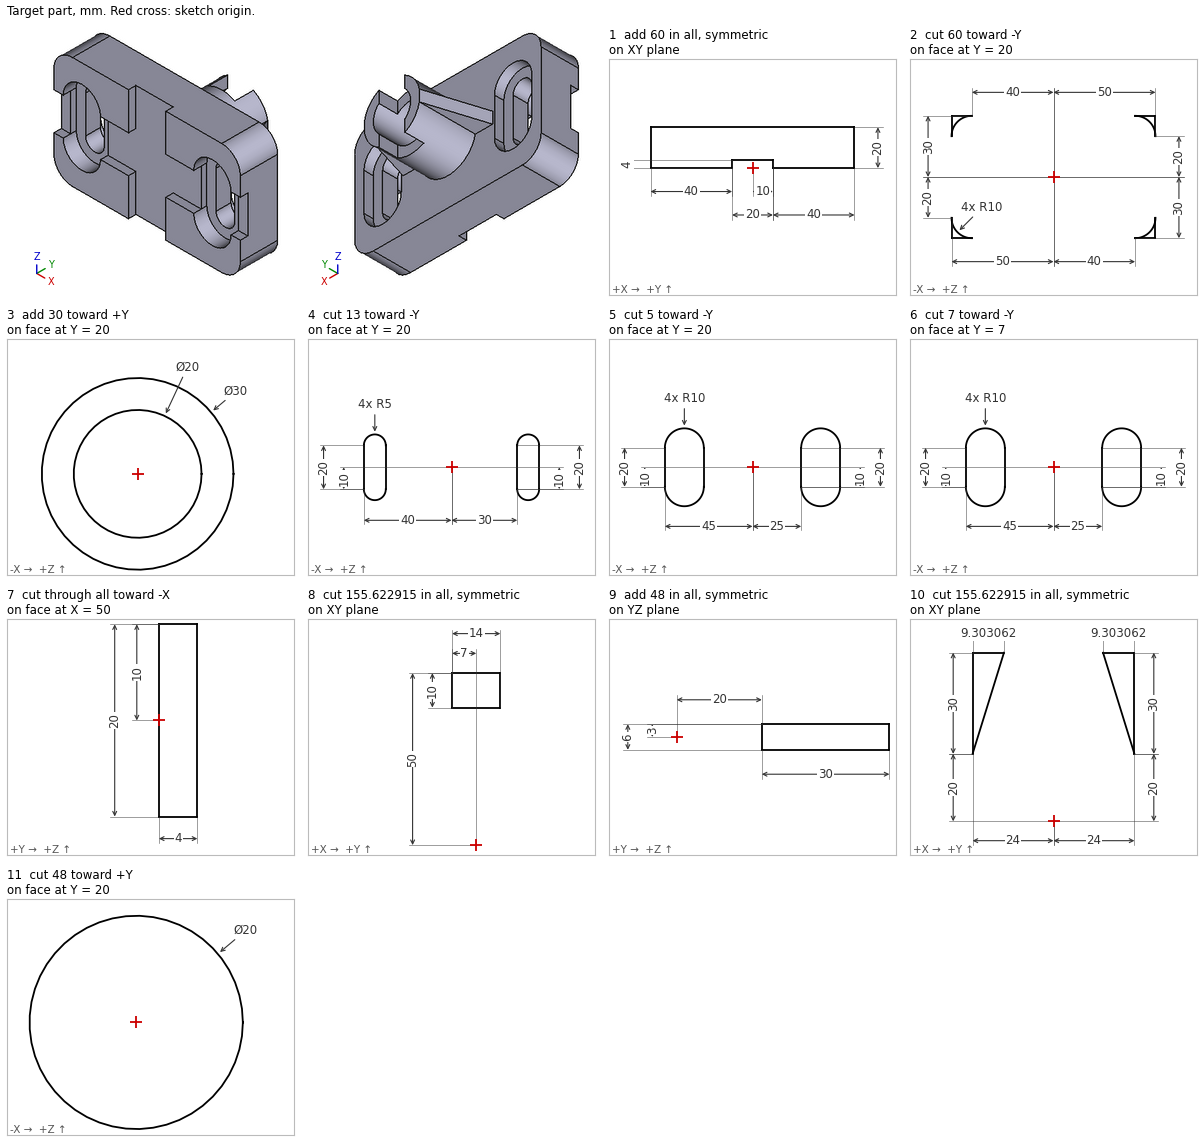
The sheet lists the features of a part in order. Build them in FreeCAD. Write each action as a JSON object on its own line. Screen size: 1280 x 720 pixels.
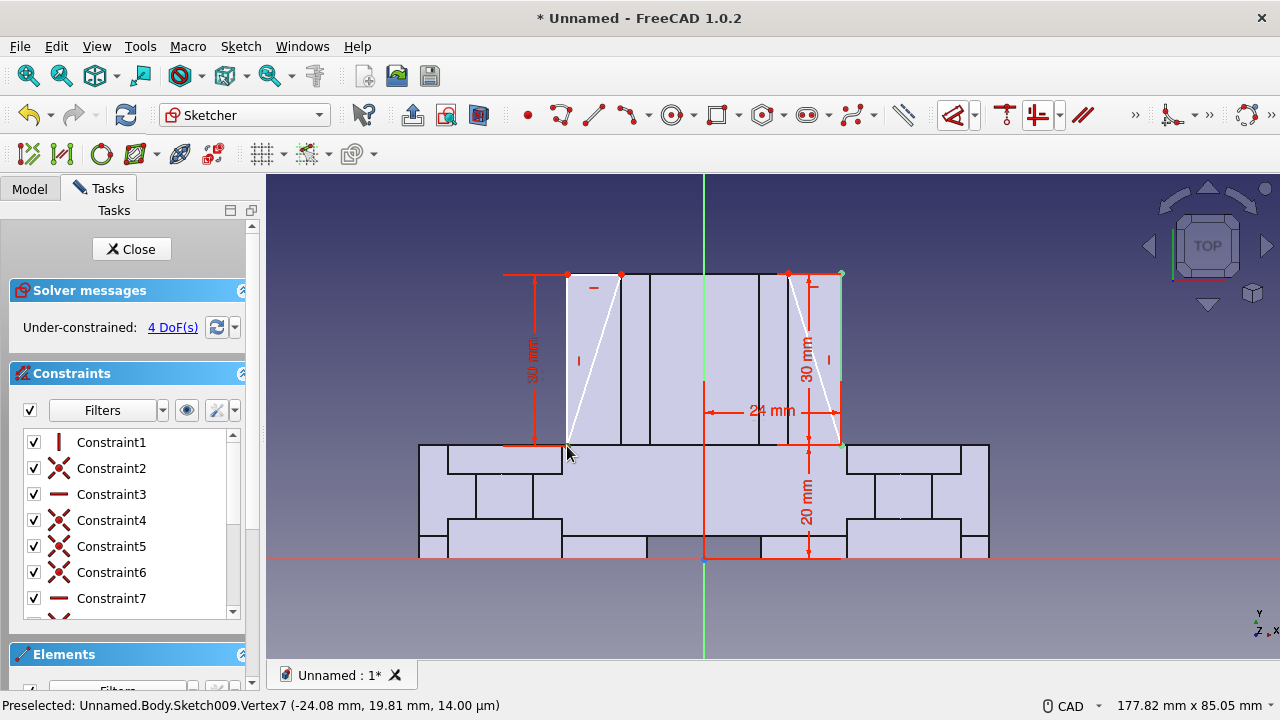
{"action": "key", "text": "l"}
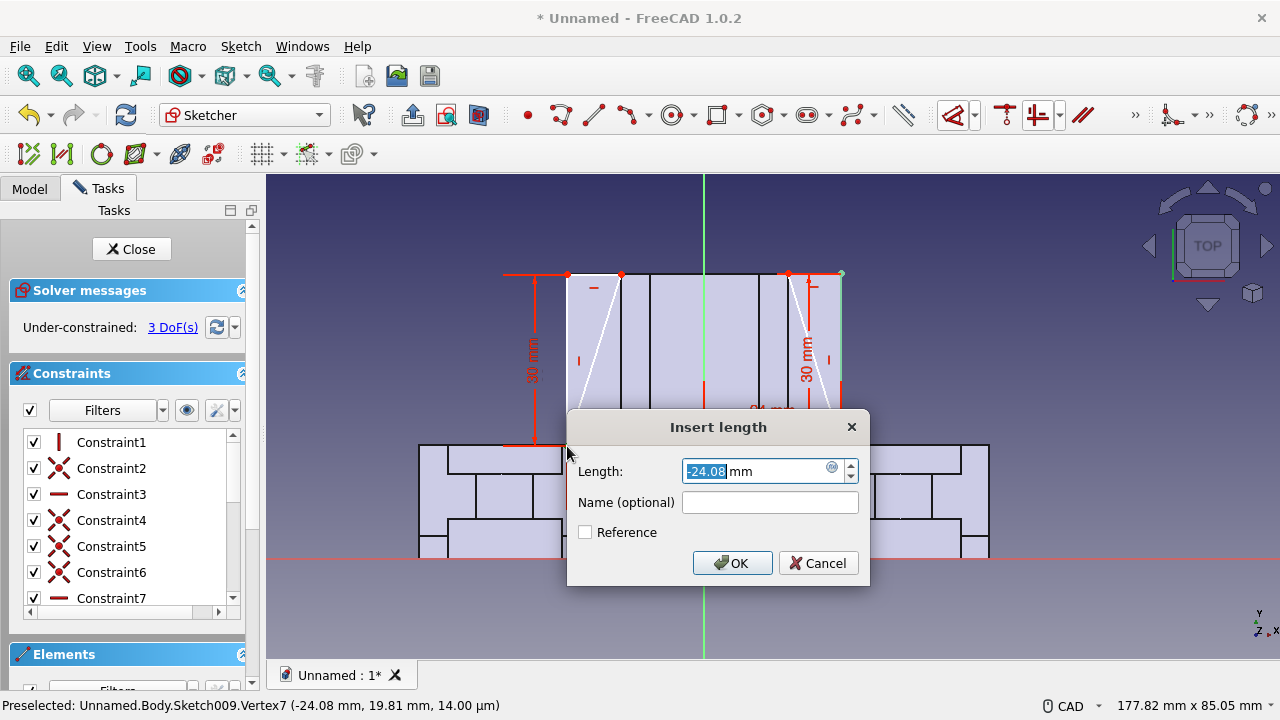
{"action": "type", "text": "-24"}
{"action": "key", "text": "Return"}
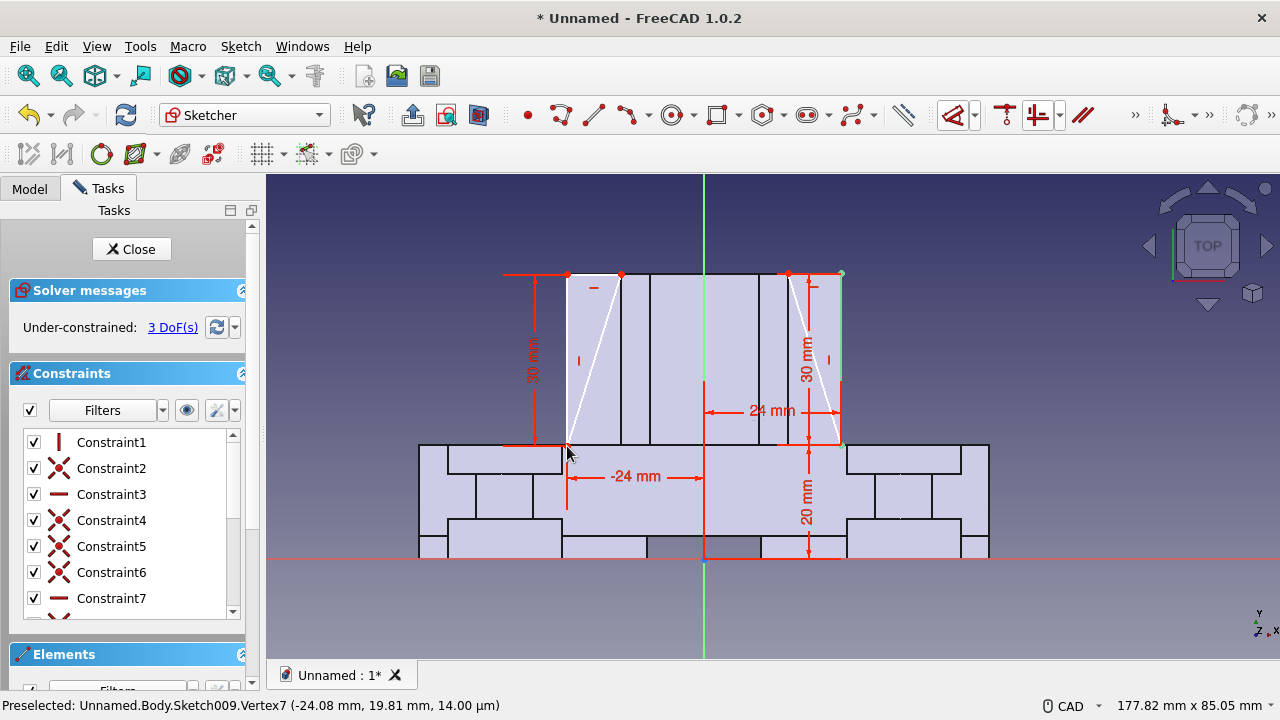
{"action": "left_click", "coordinate": [567, 446]}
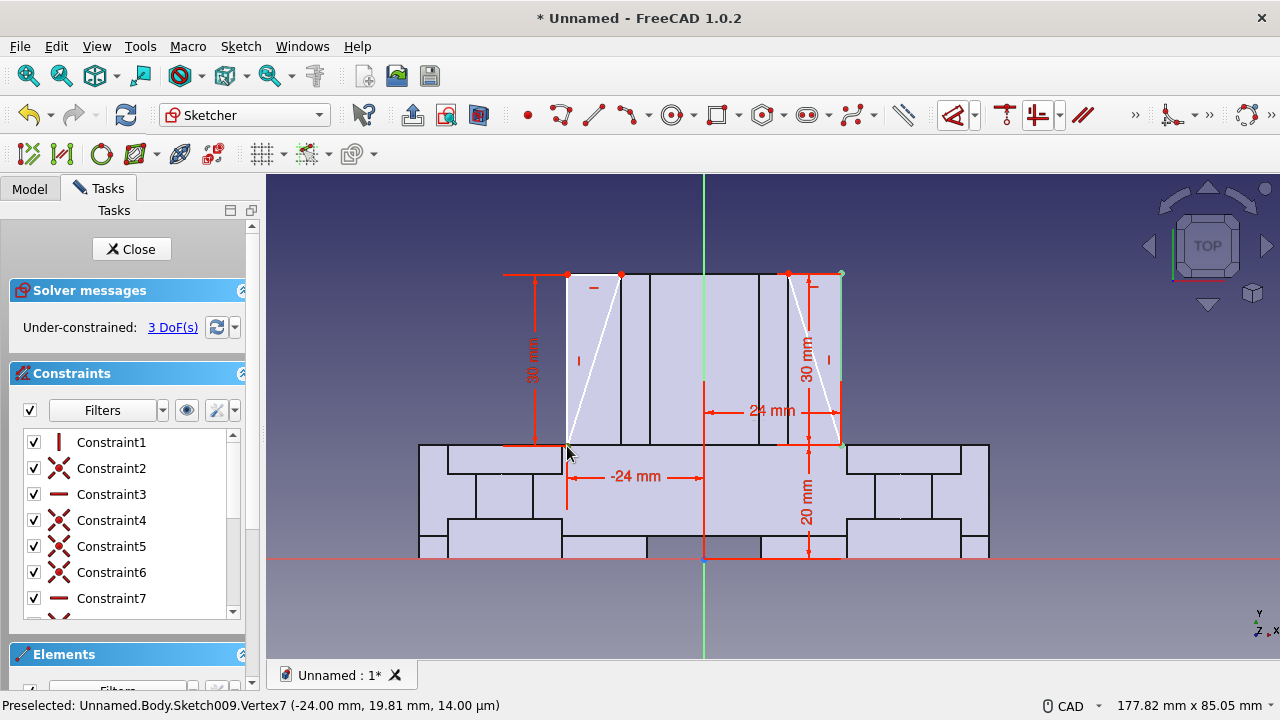
{"action": "key", "text": "i"}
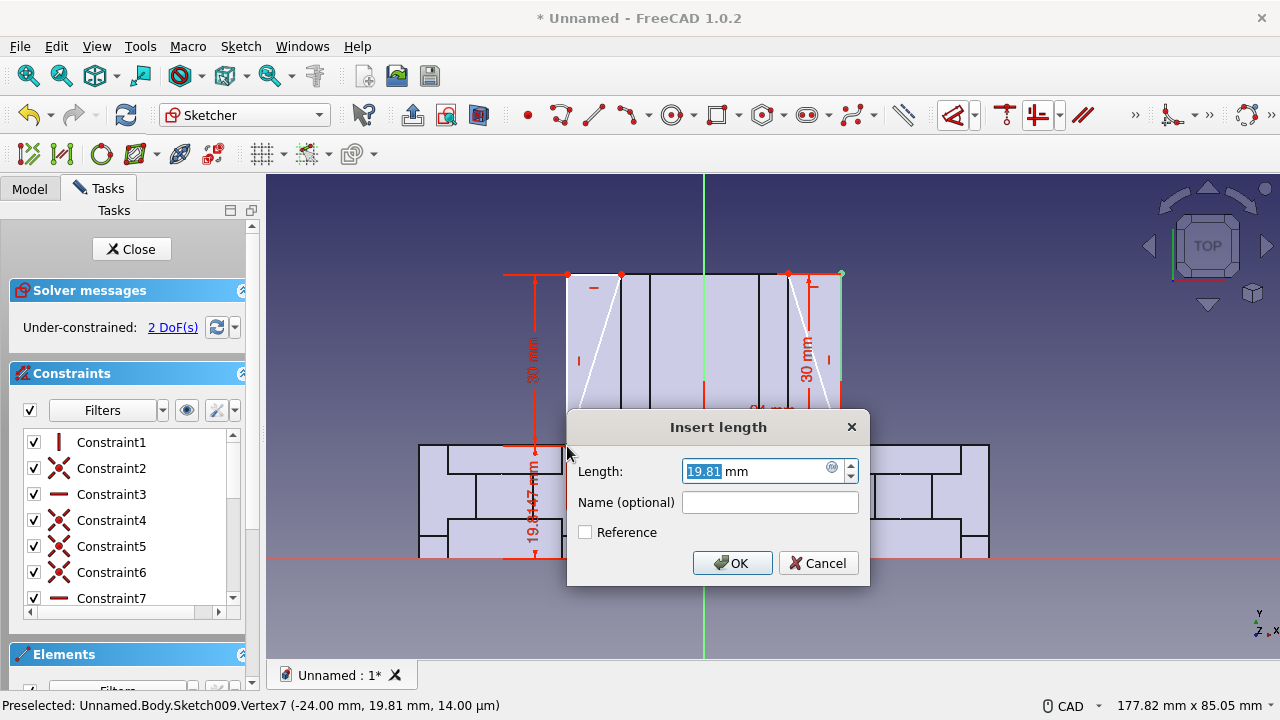
{"action": "type", "text": "20"}
{"action": "key", "text": "Return"}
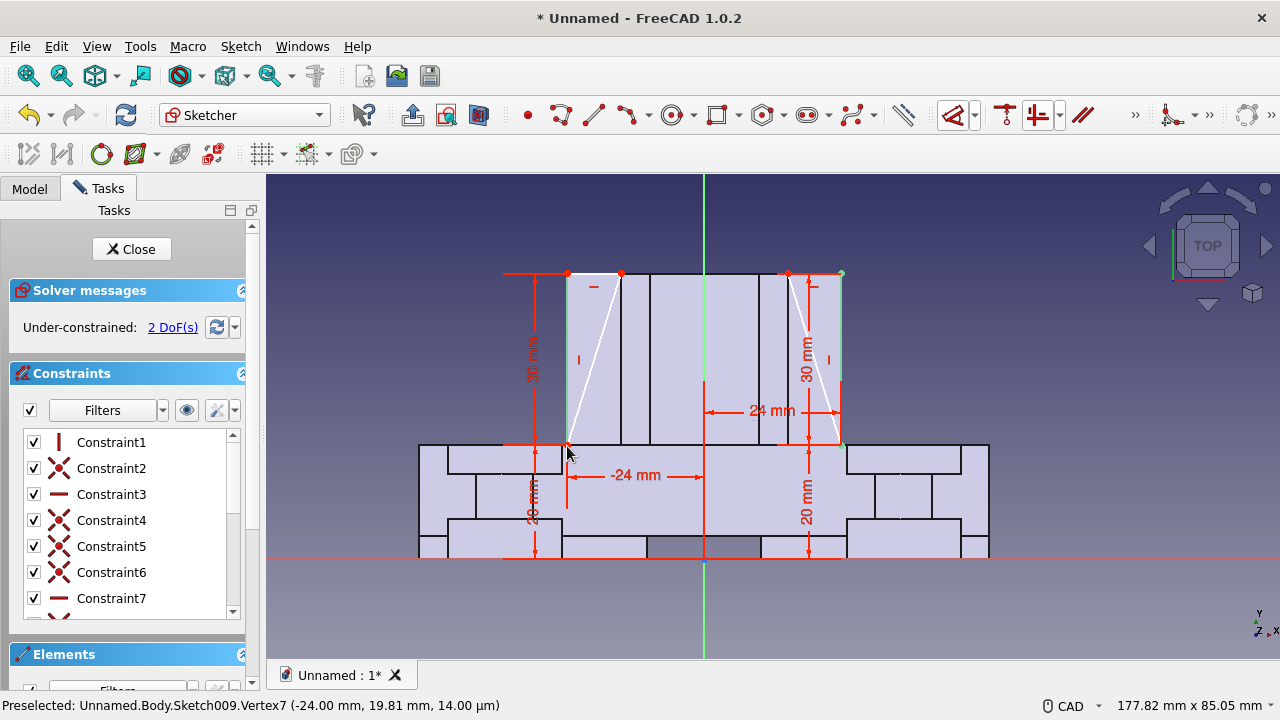
{"action": "left_click", "coordinate": [825, 274]}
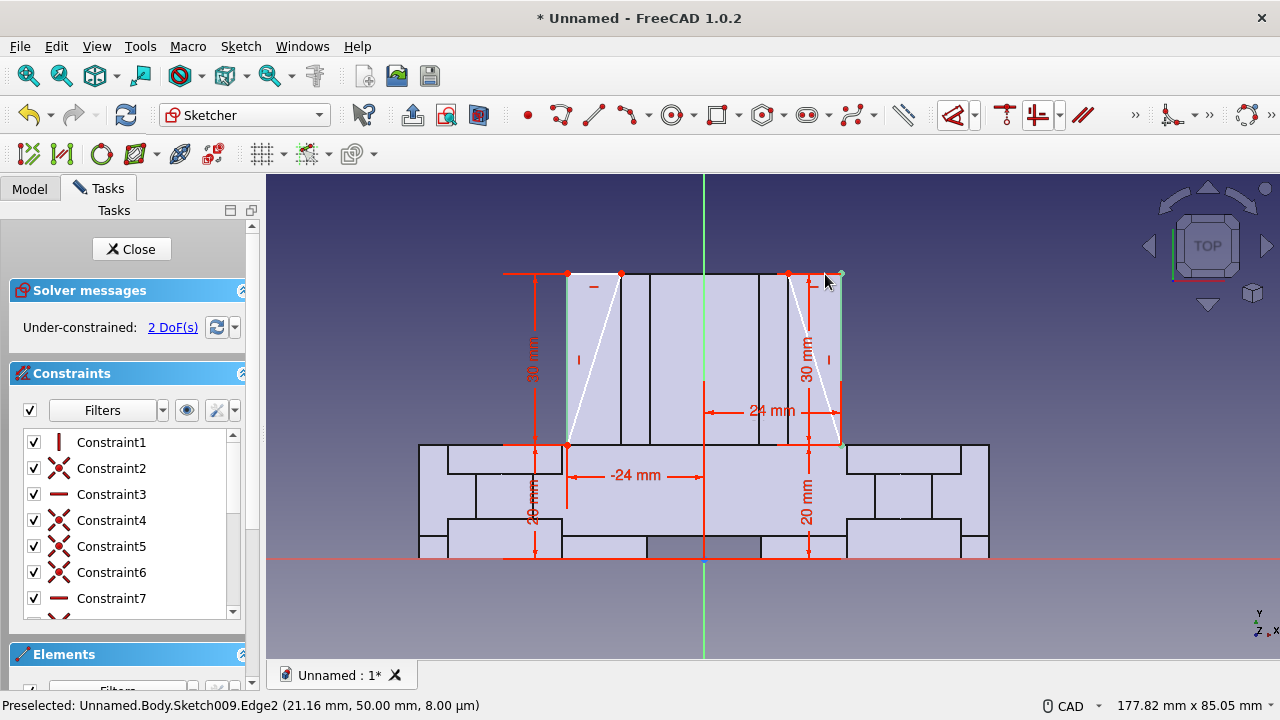
{"action": "key", "text": "l"}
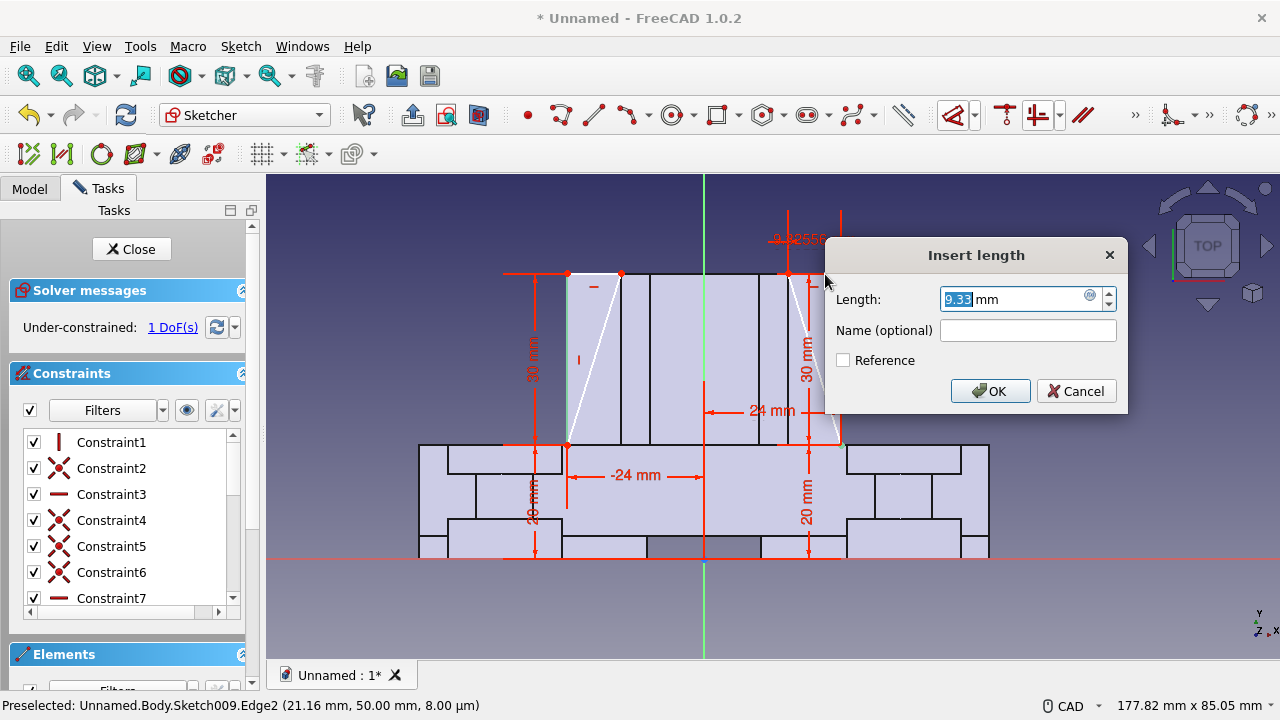
{"action": "type", "text": "9.303062"}
{"action": "key", "text": "Return"}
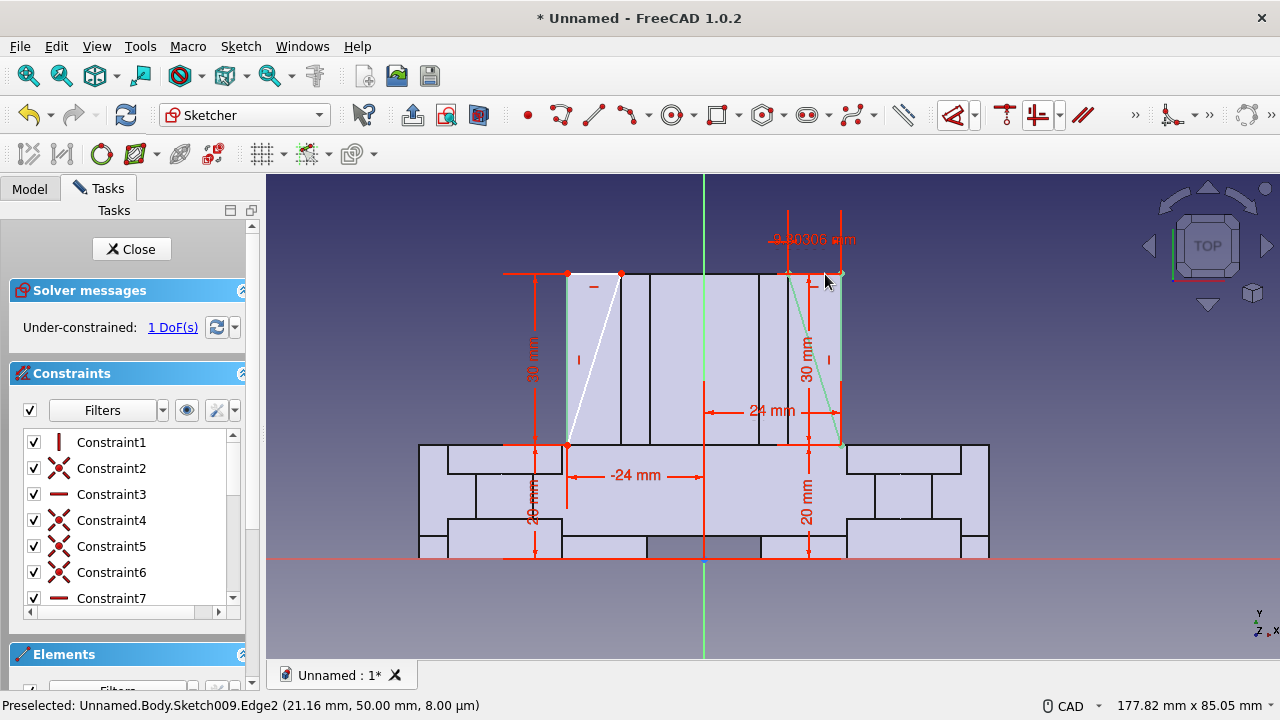
{"action": "left_click", "coordinate": [605, 274]}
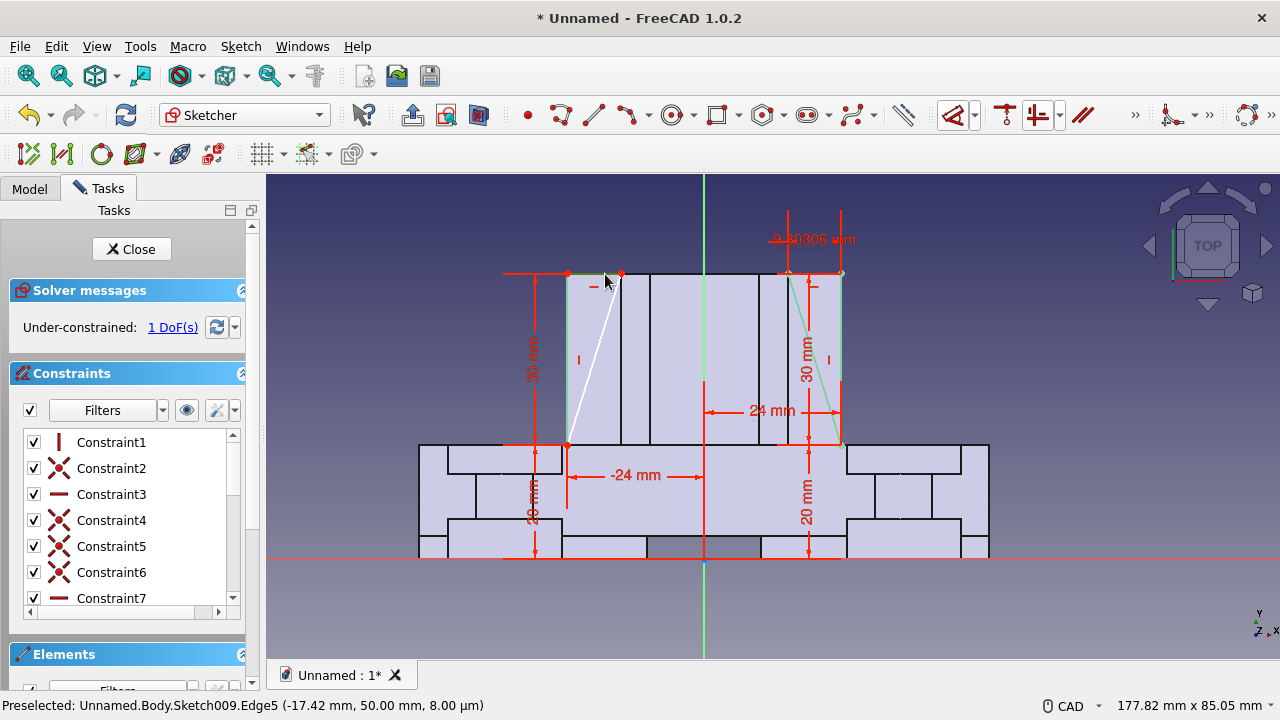
{"action": "key", "text": "l"}